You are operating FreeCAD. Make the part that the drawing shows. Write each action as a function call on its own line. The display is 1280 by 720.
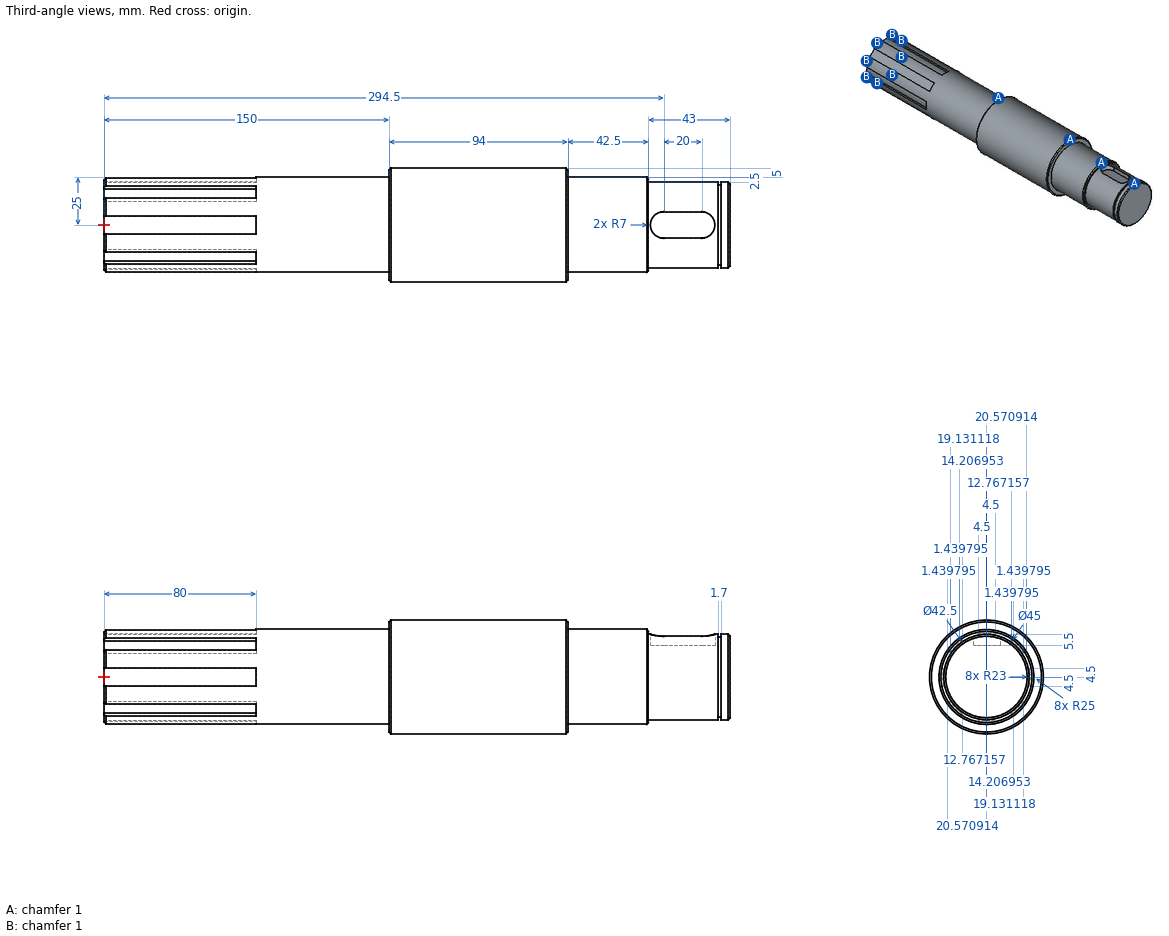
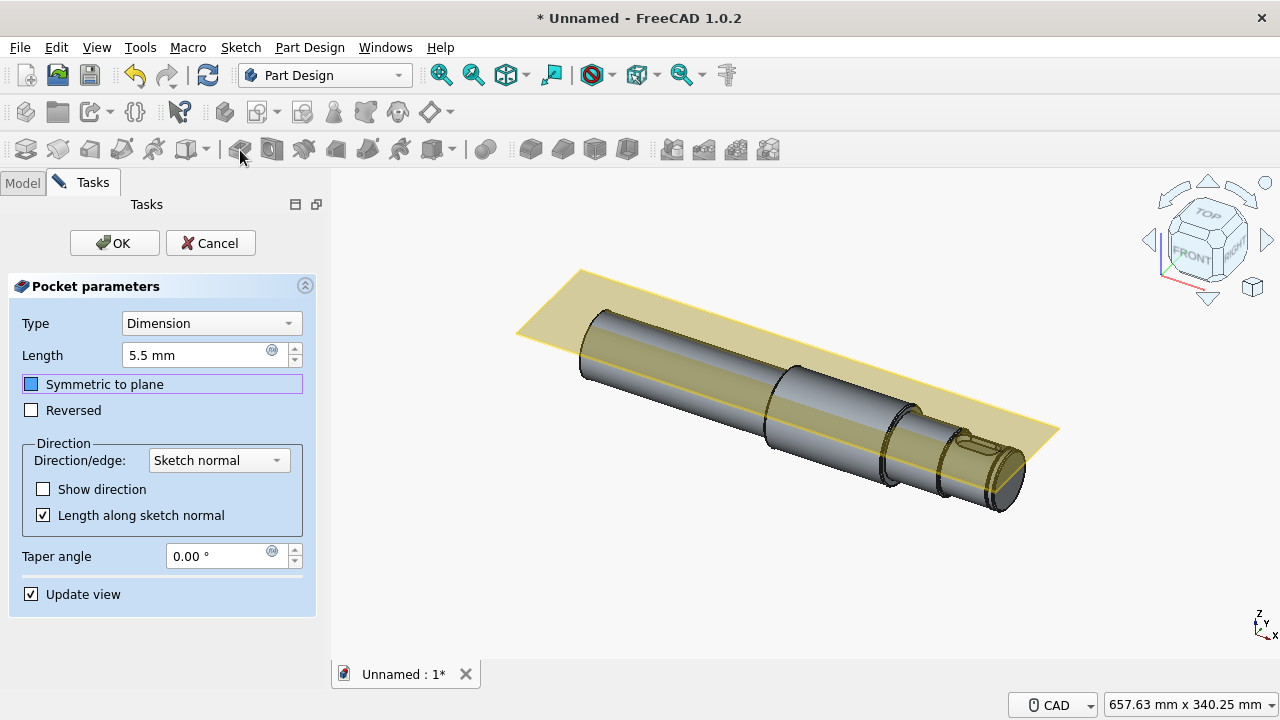
click(115, 243)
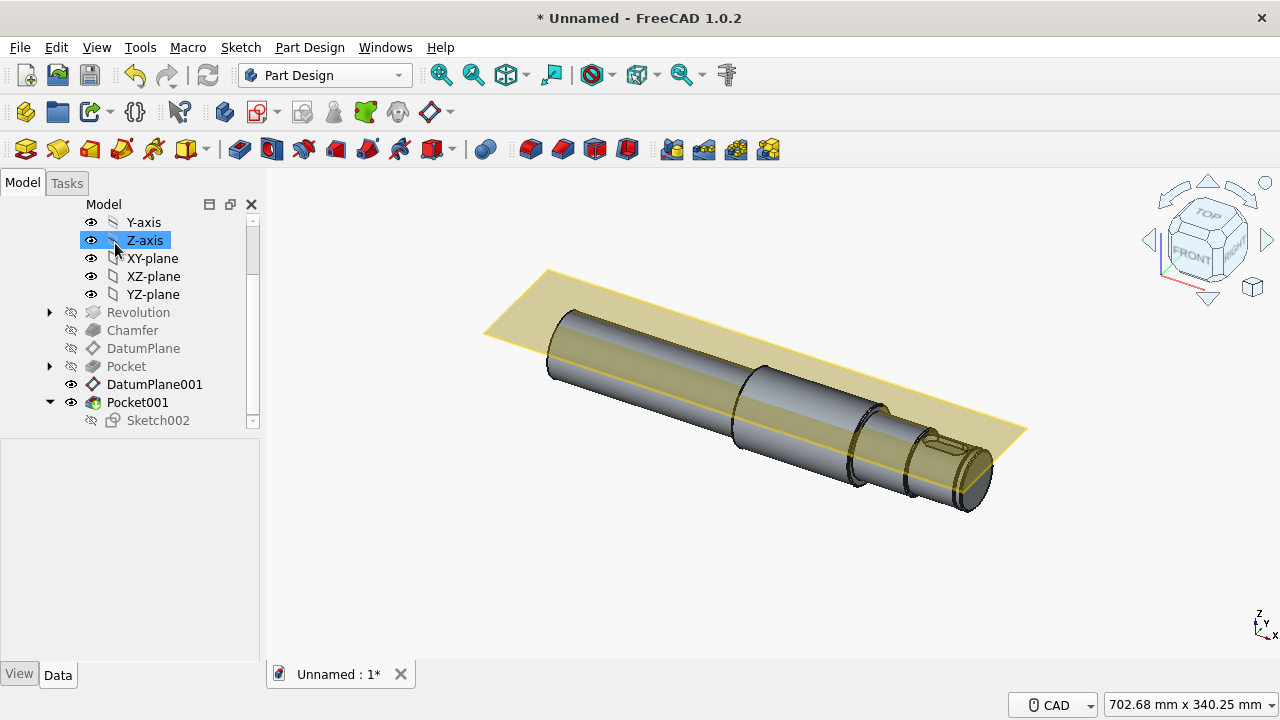
click(116, 384)
key(space)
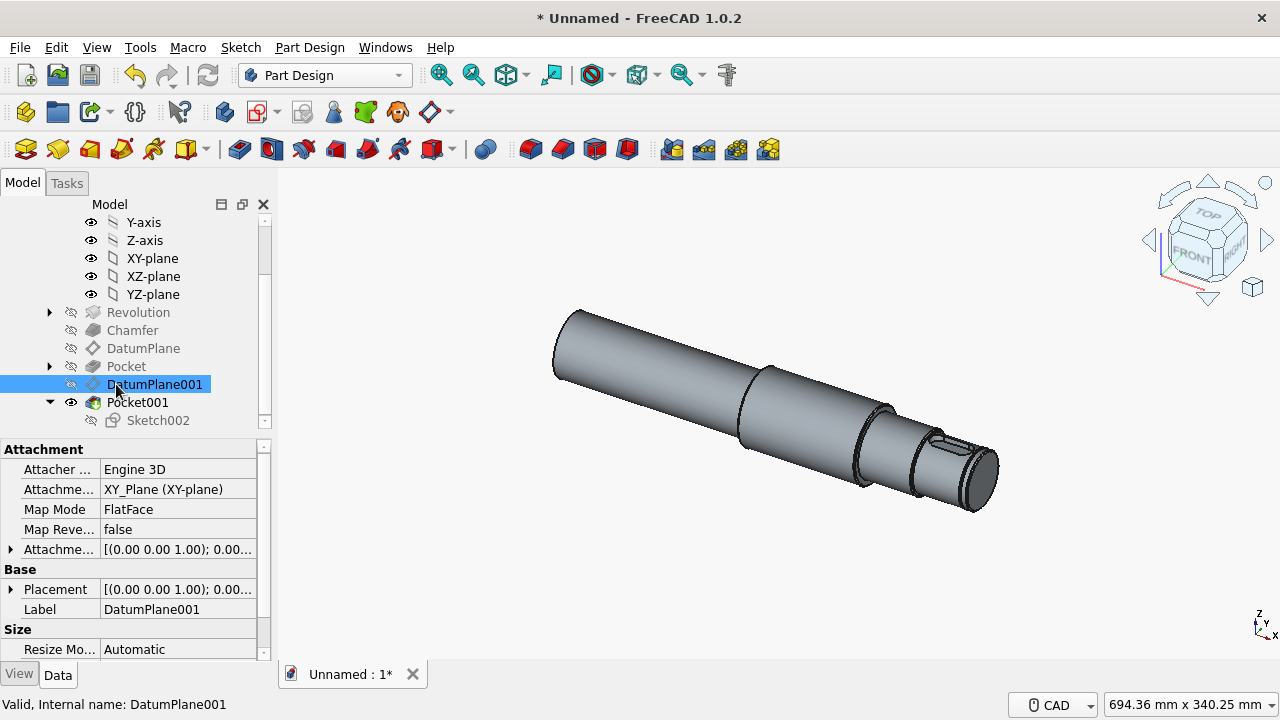
scroll(160, 326, down, 3)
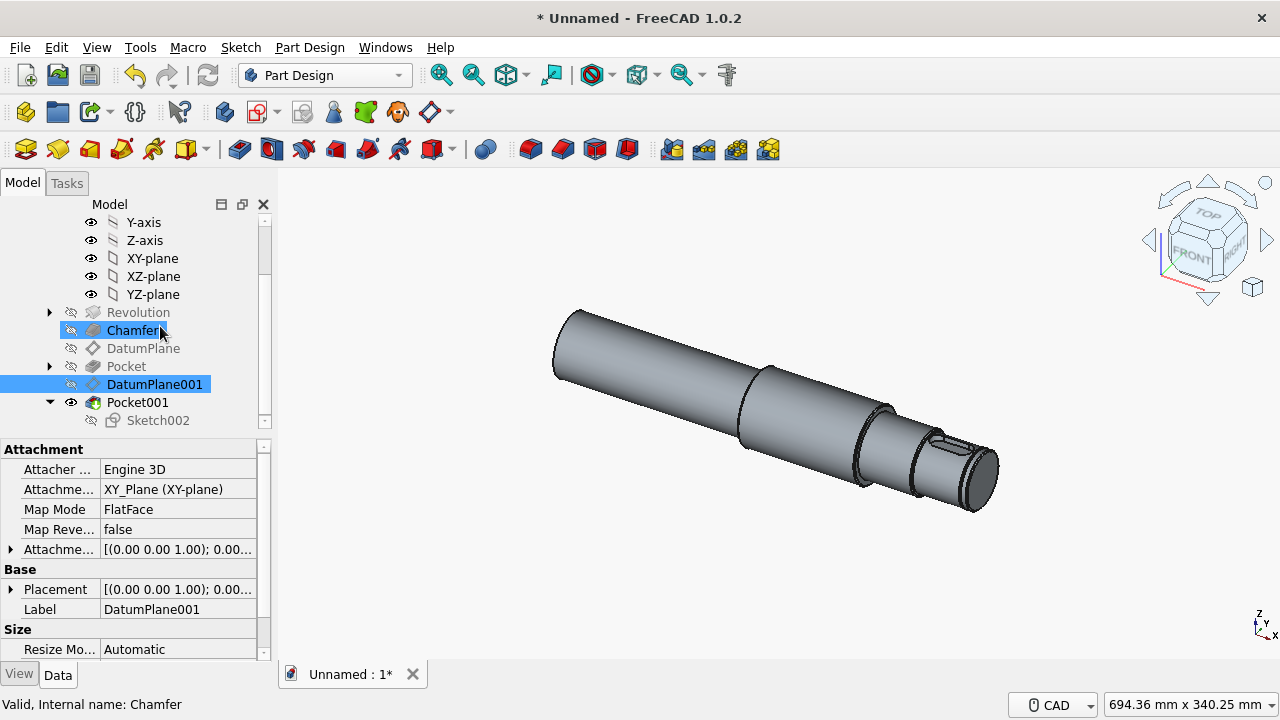
scroll(160, 326, up, 15)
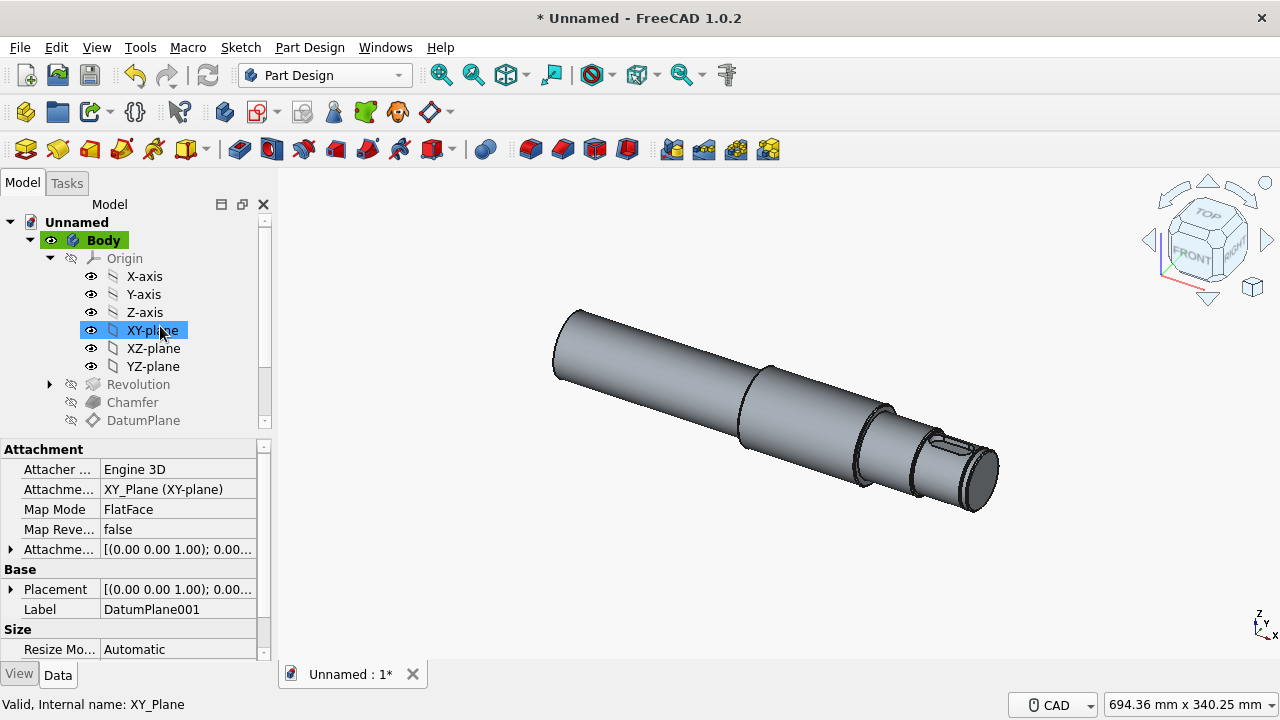
click(136, 366)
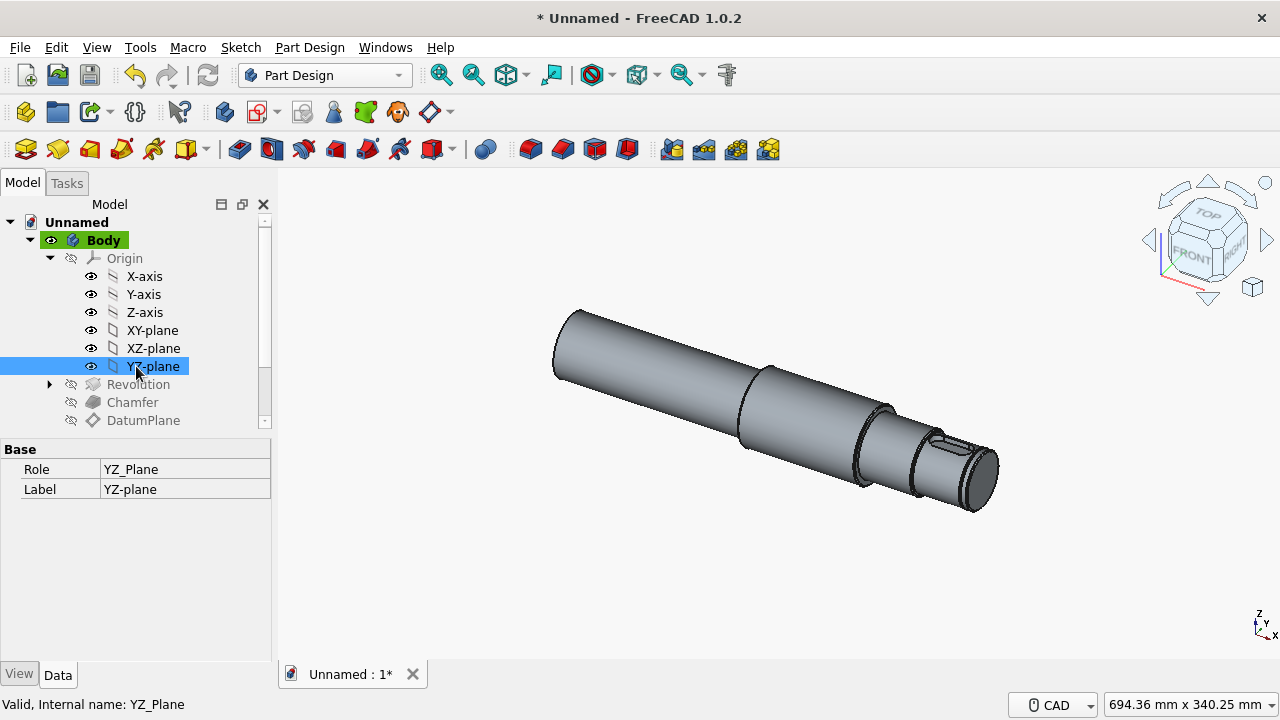
click(430, 112)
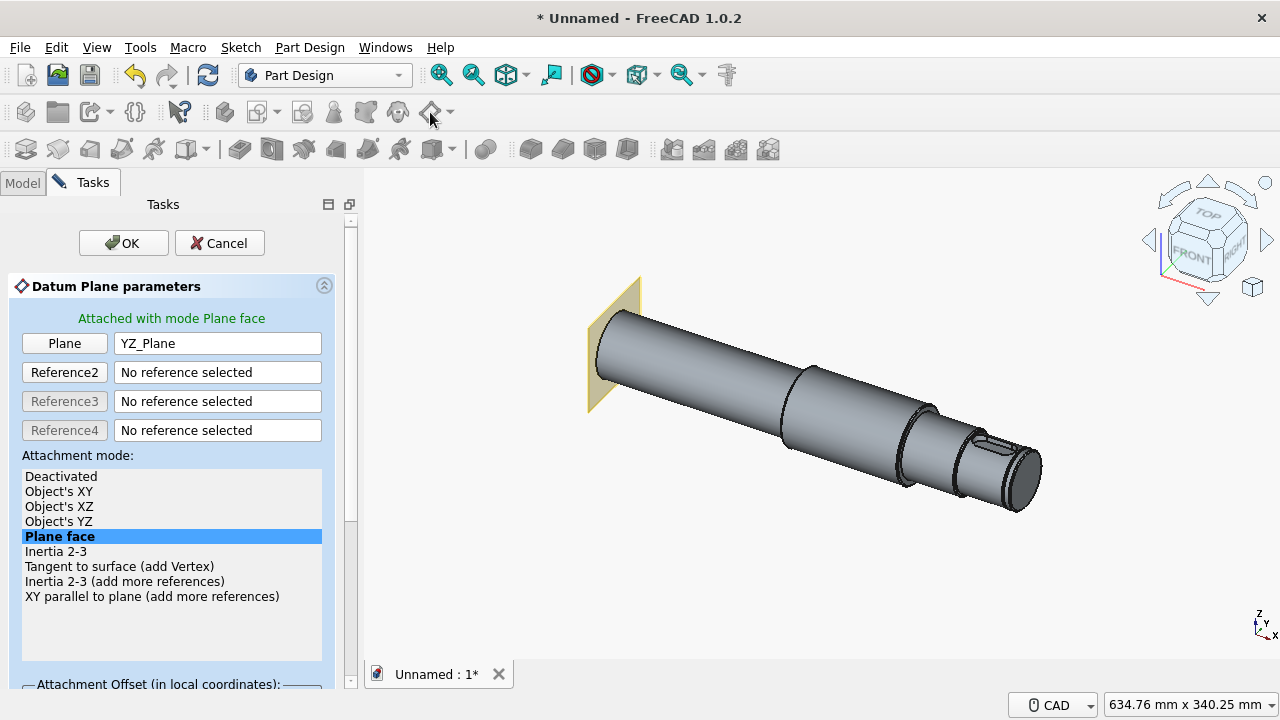
scroll(351, 451, down, 3)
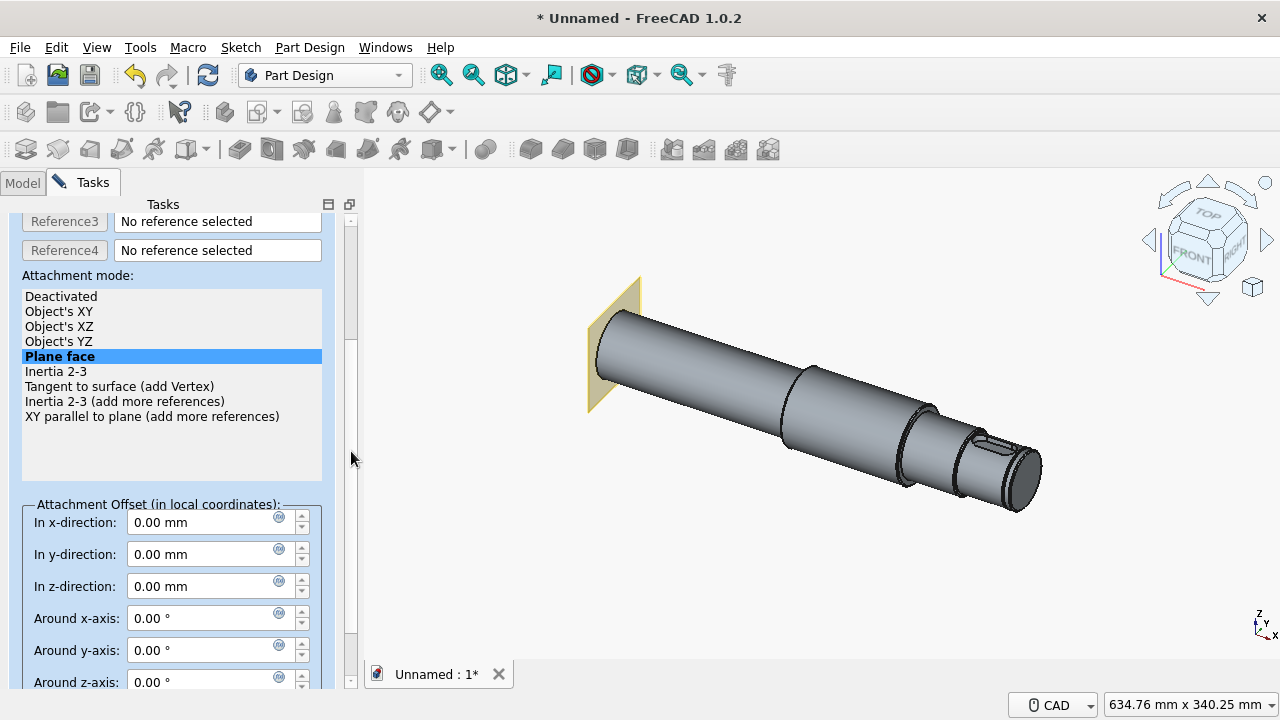
triple_click(210, 586)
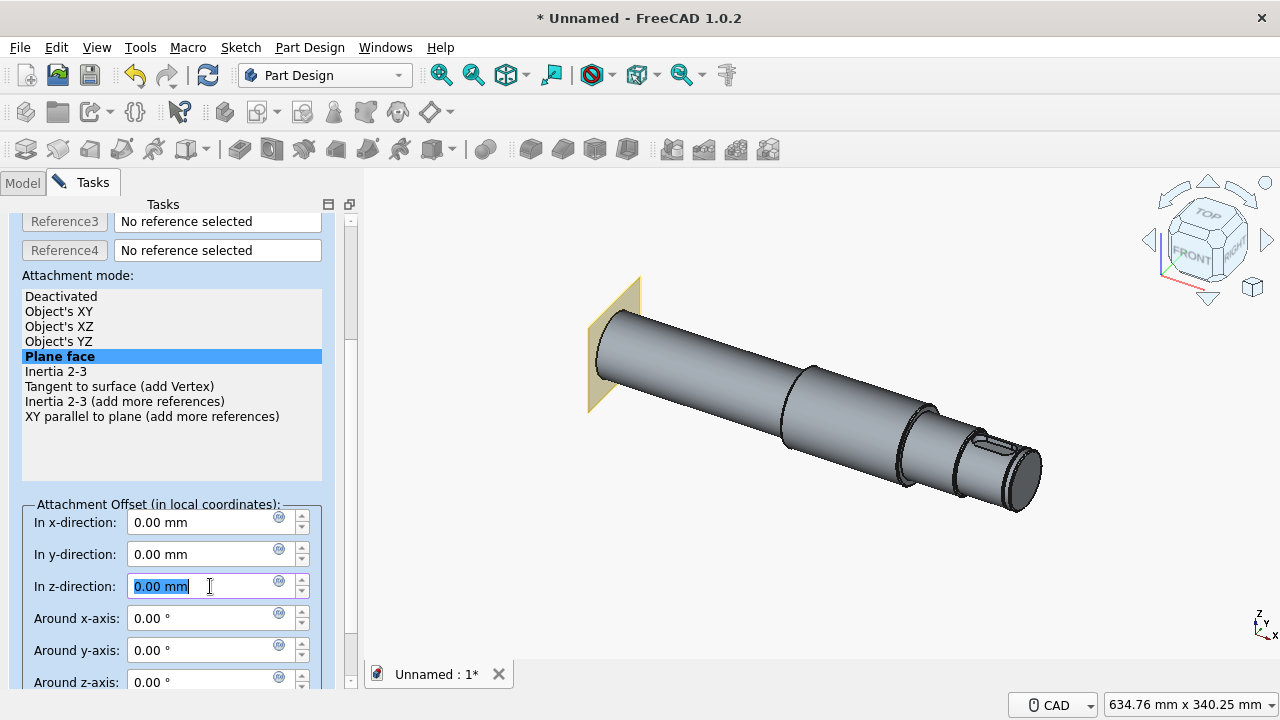
text(80)
key(Tab)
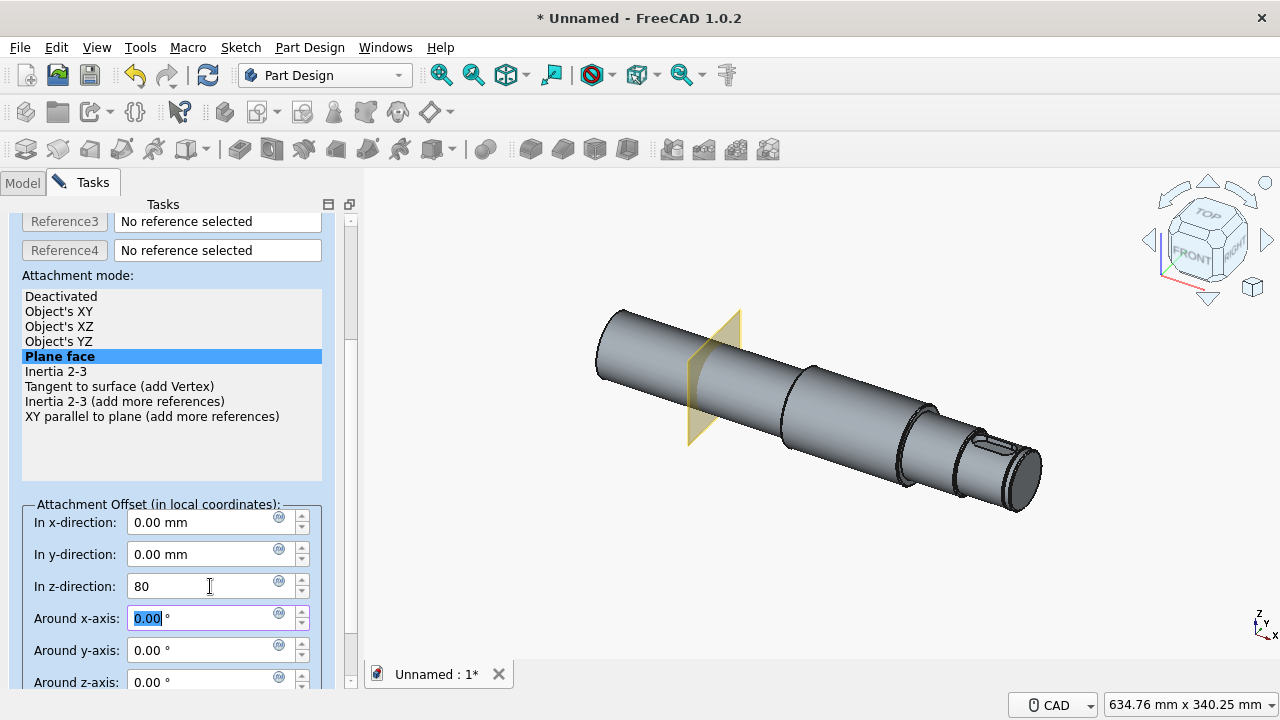
scroll(351, 451, up, 4)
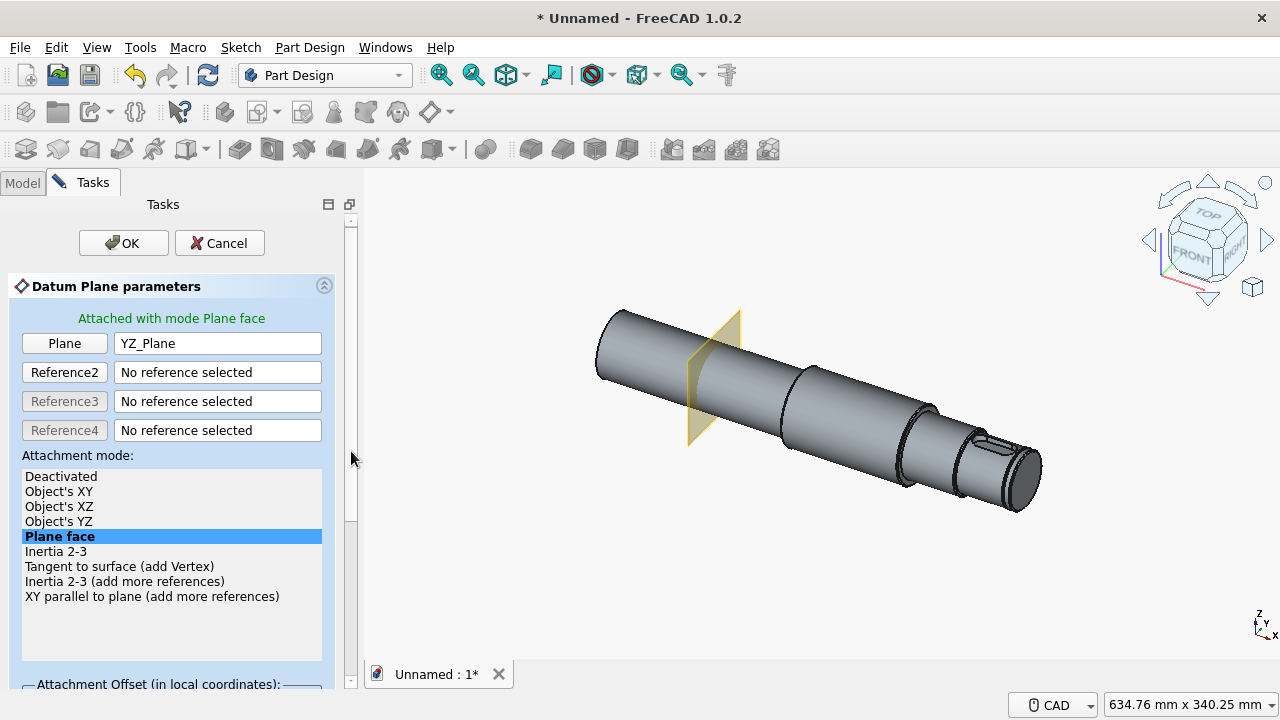
click(124, 243)